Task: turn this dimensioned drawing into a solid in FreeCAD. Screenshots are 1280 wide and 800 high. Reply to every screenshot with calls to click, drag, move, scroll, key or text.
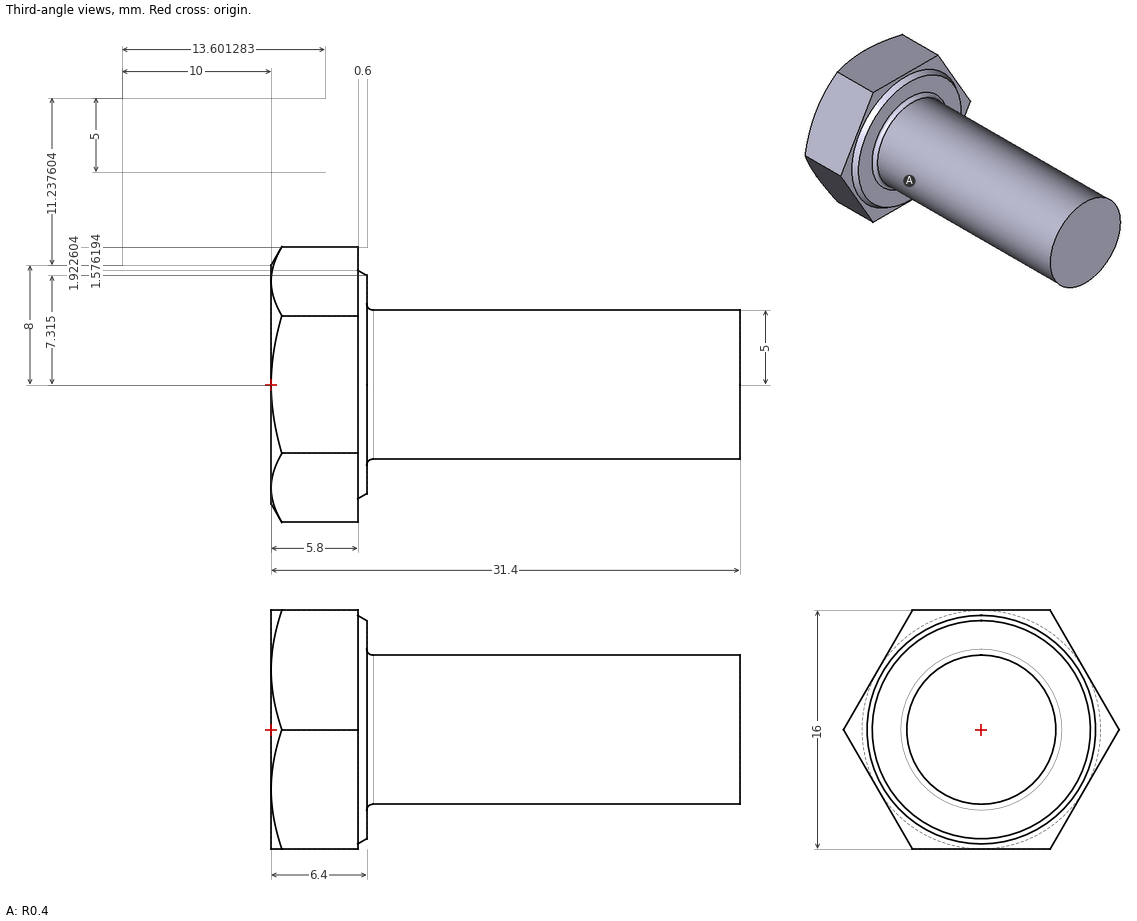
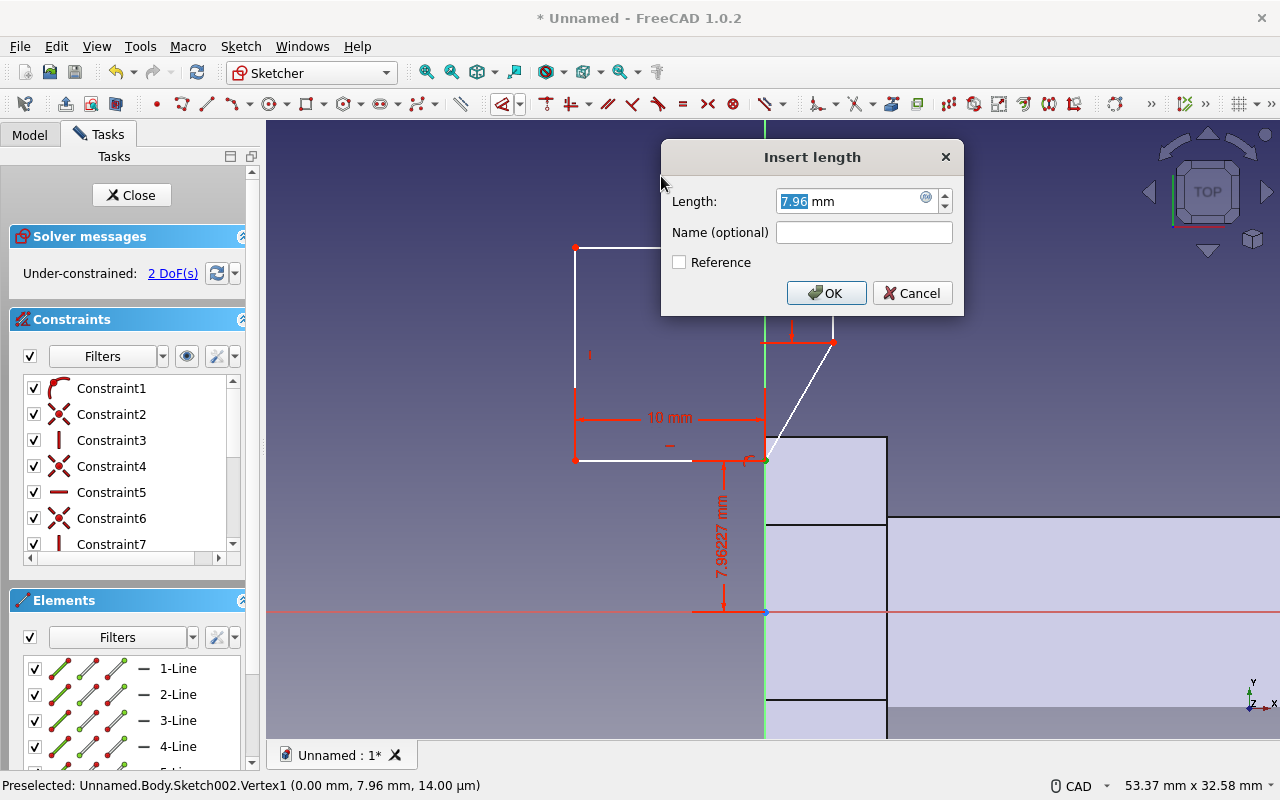
text(8)
key(Return)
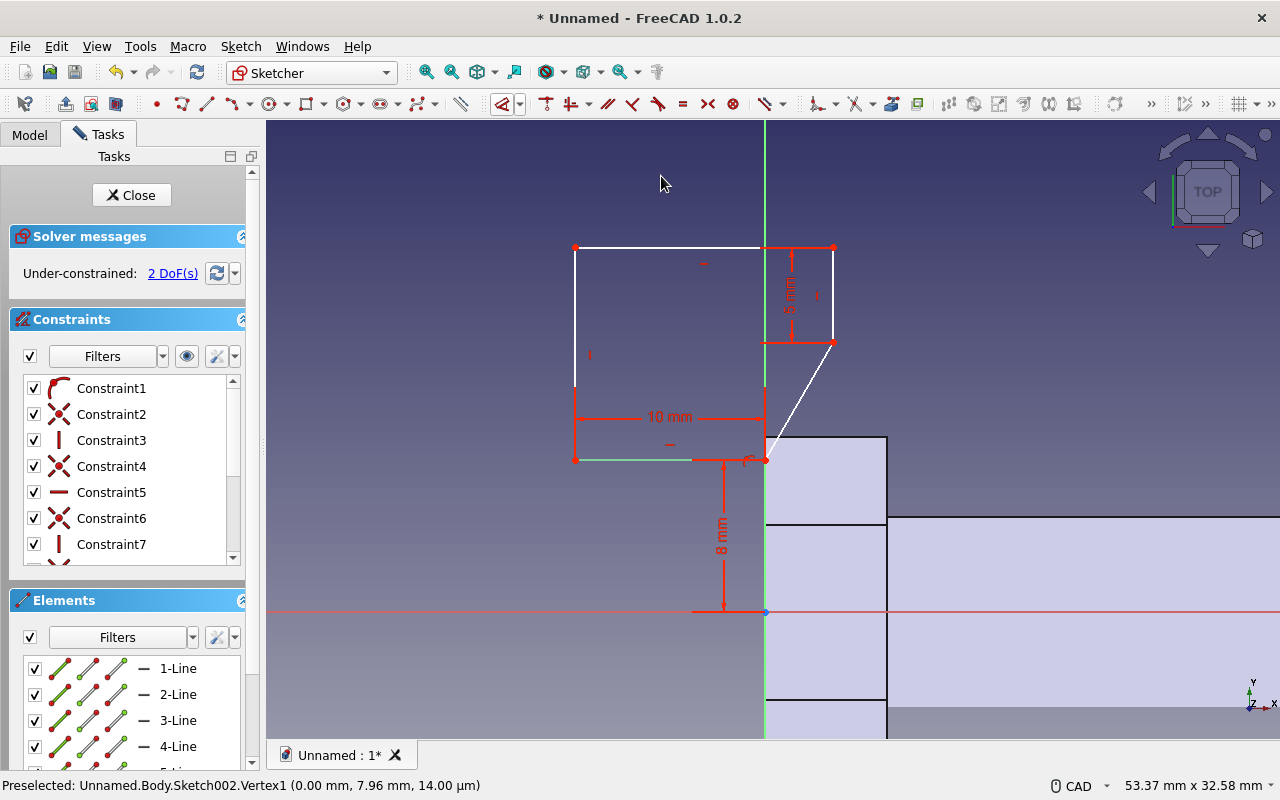
scroll(756, 248, up, 2)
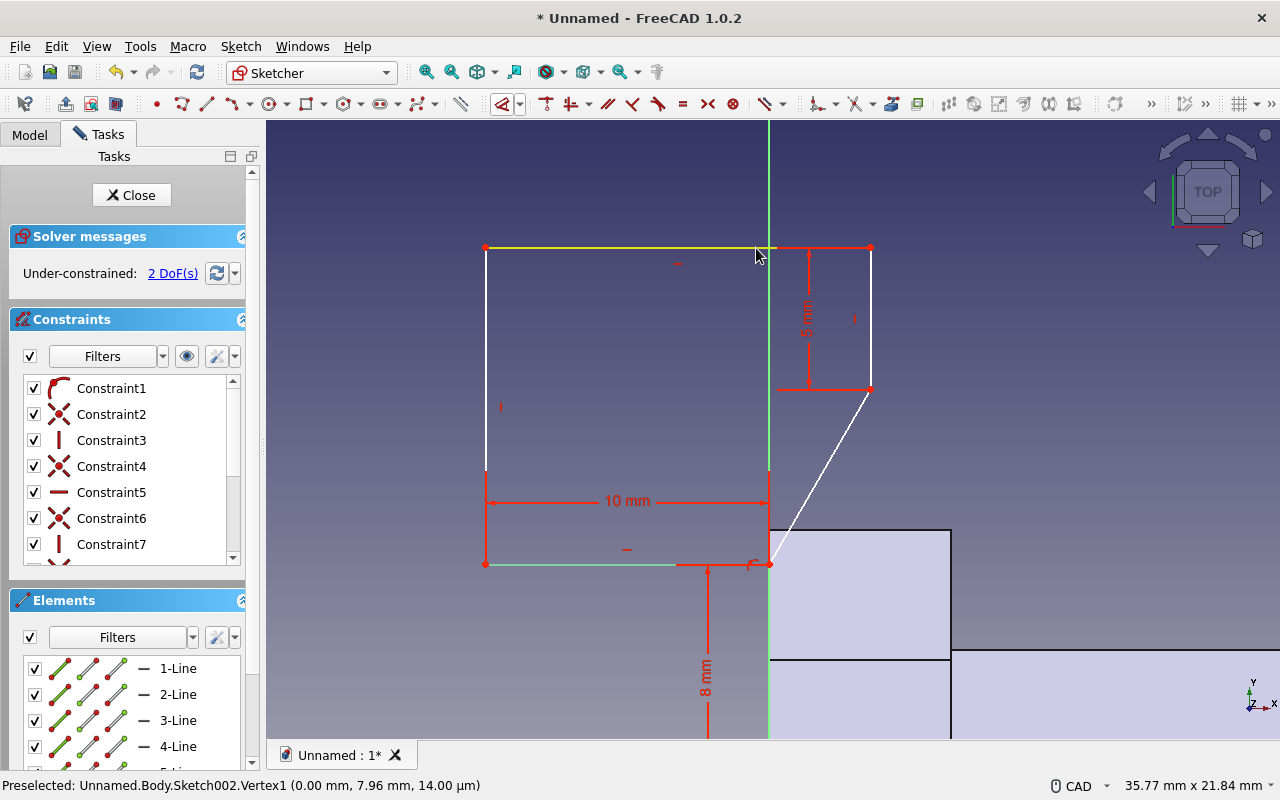
click(755, 248)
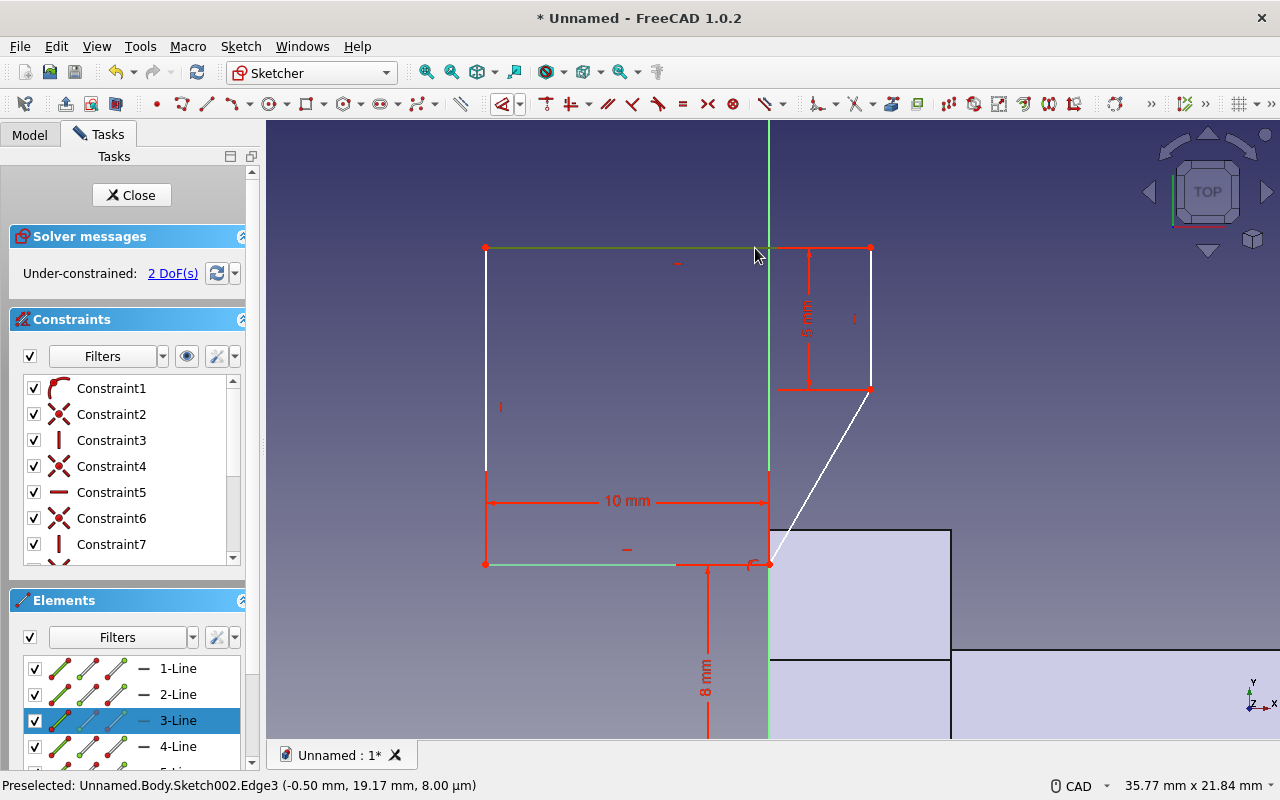
click(520, 104)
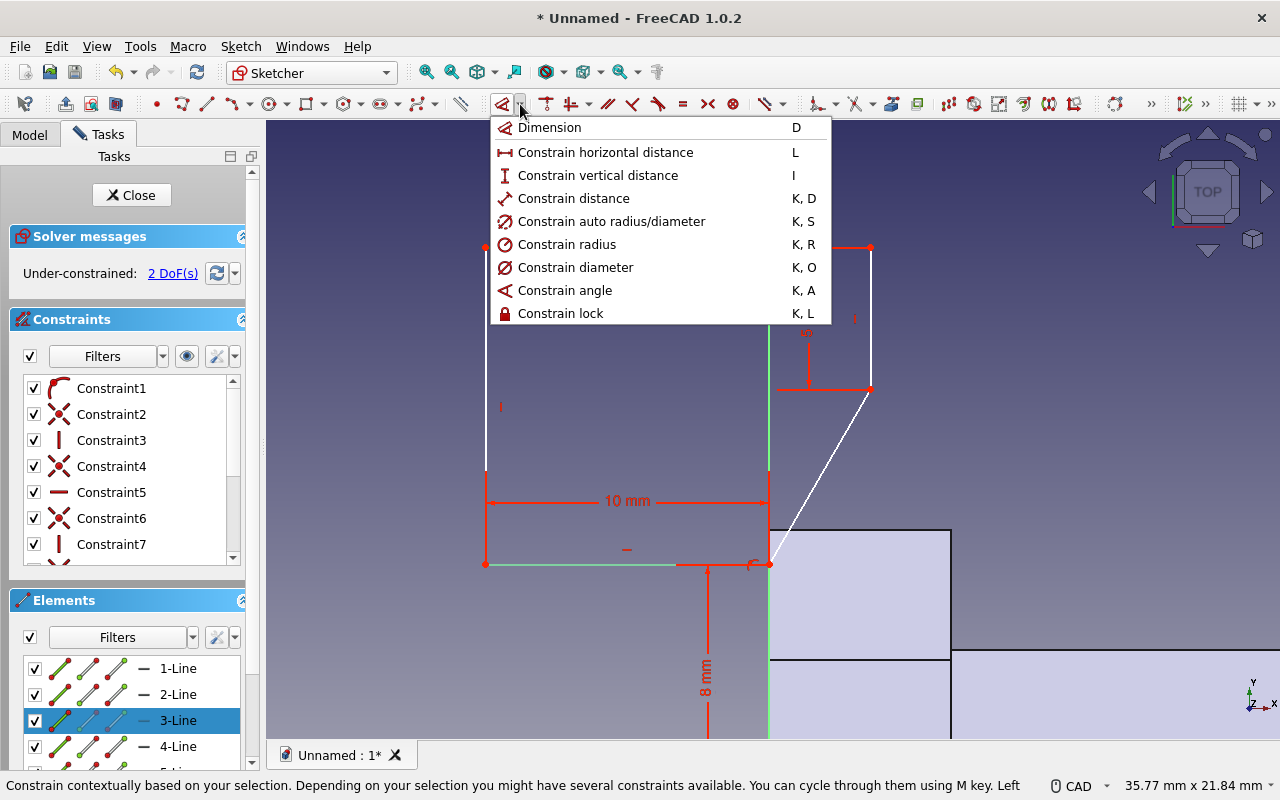
click(661, 152)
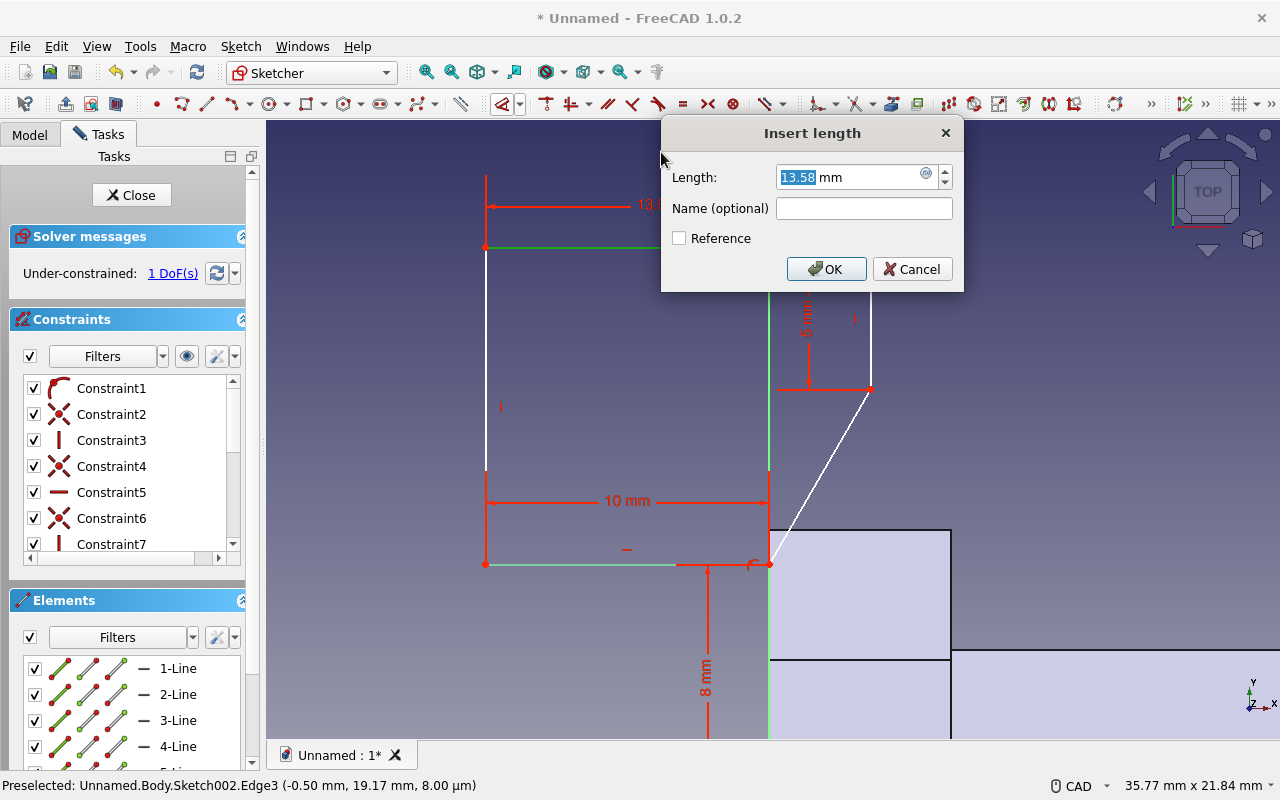
text(13.601283)
key(Return)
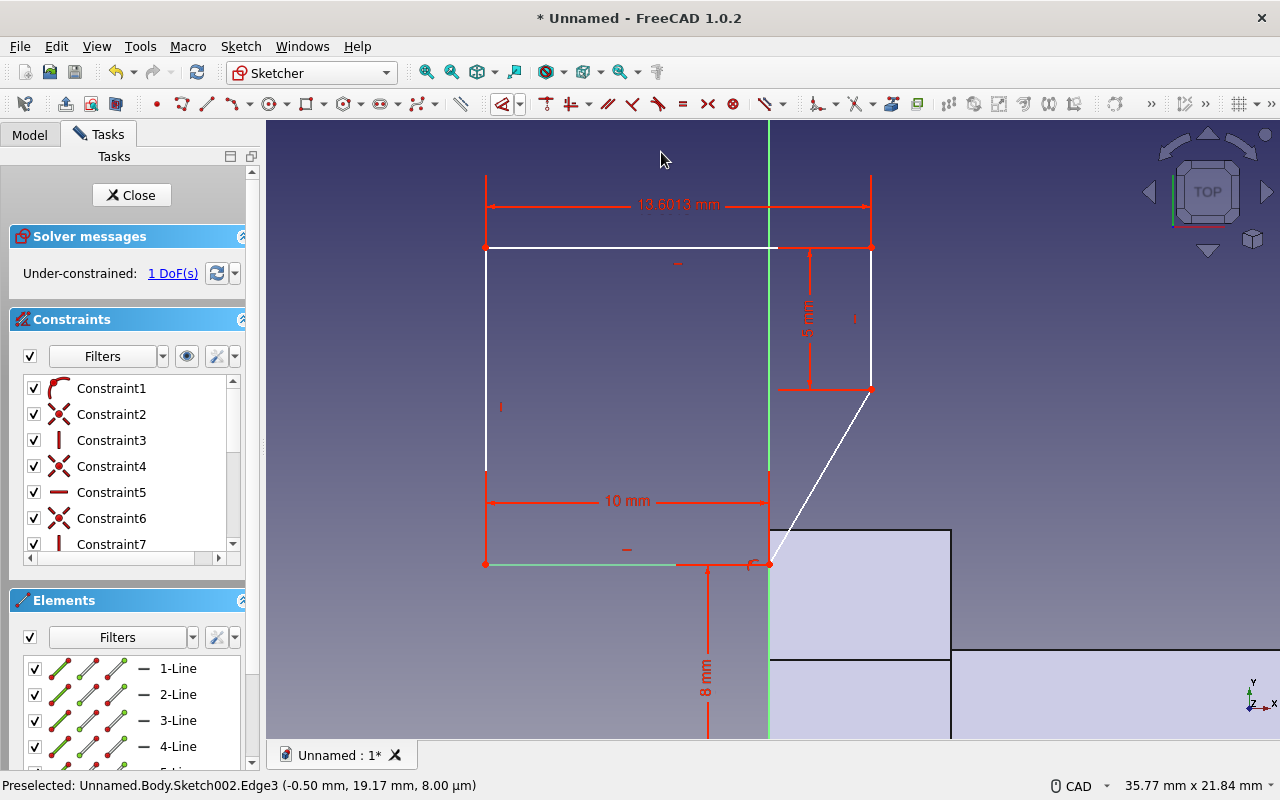
click(486, 343)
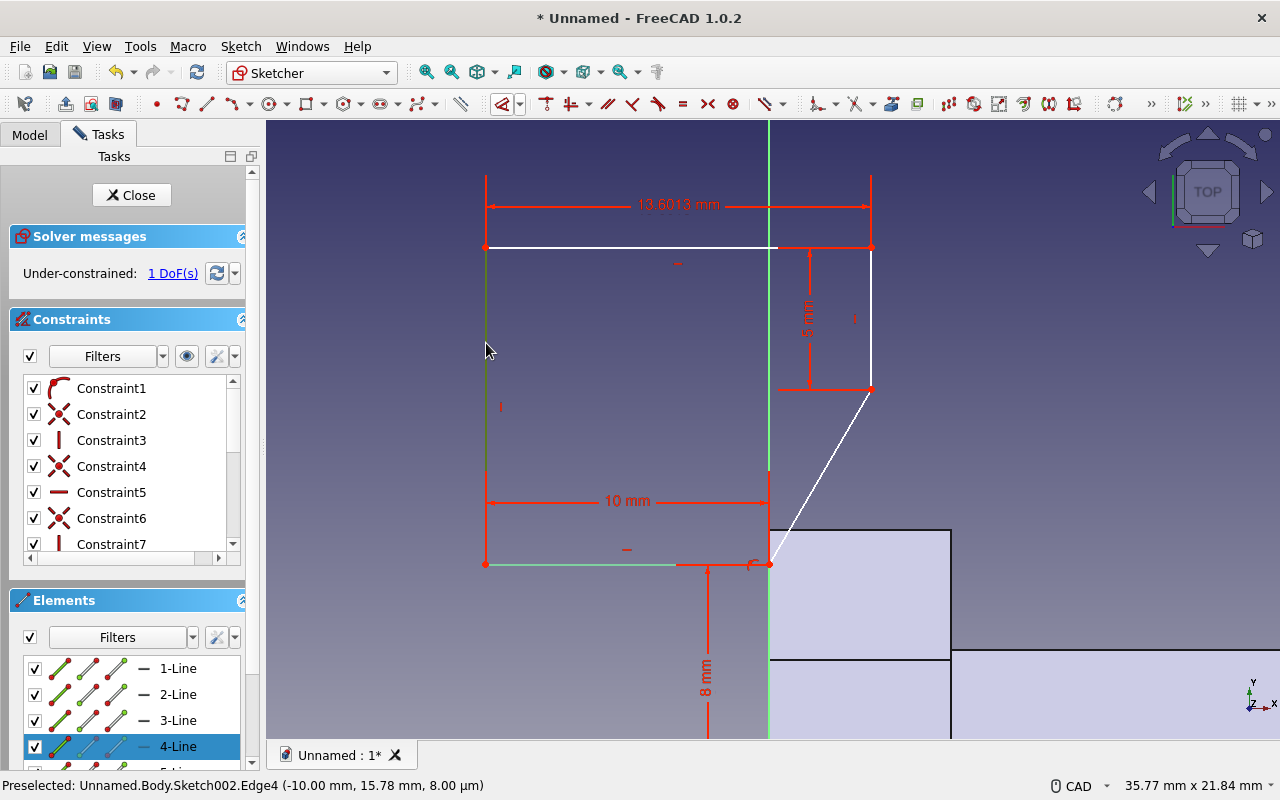
key(i)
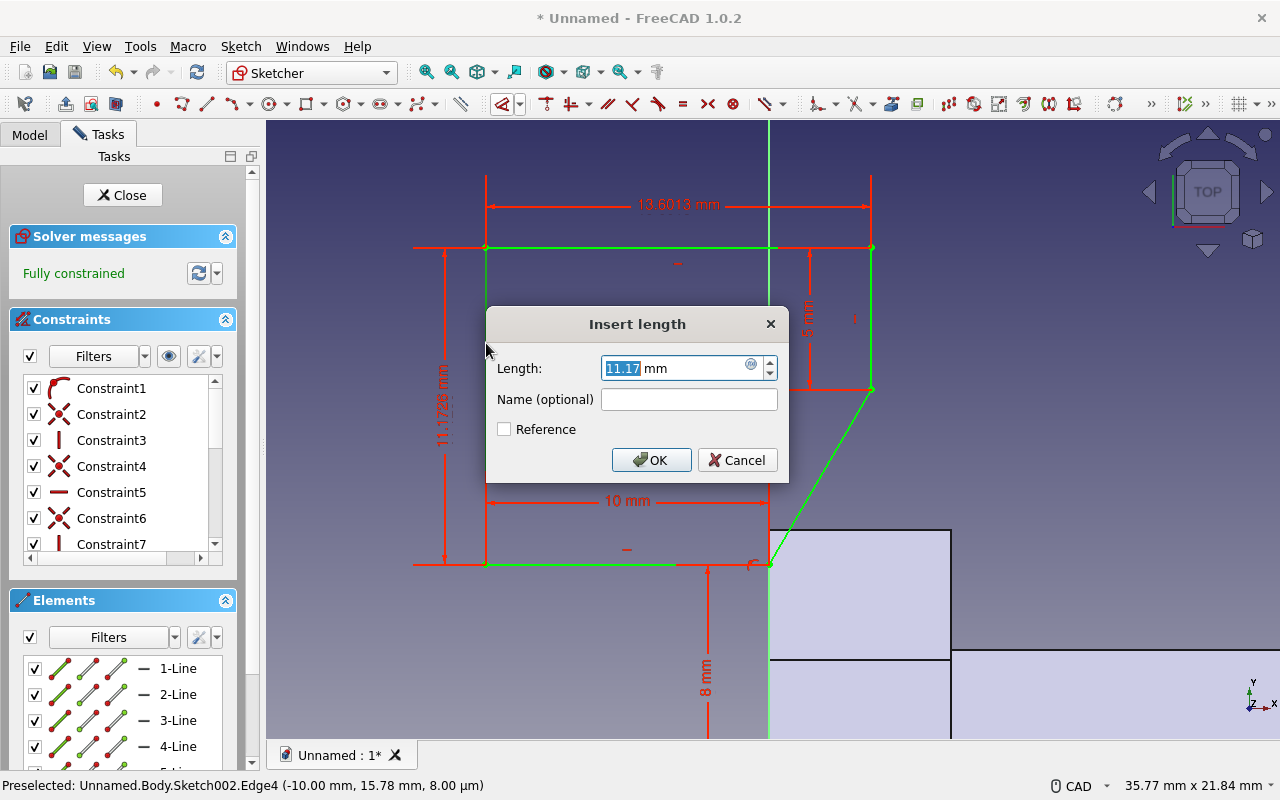
text(11.237604)
key(Return)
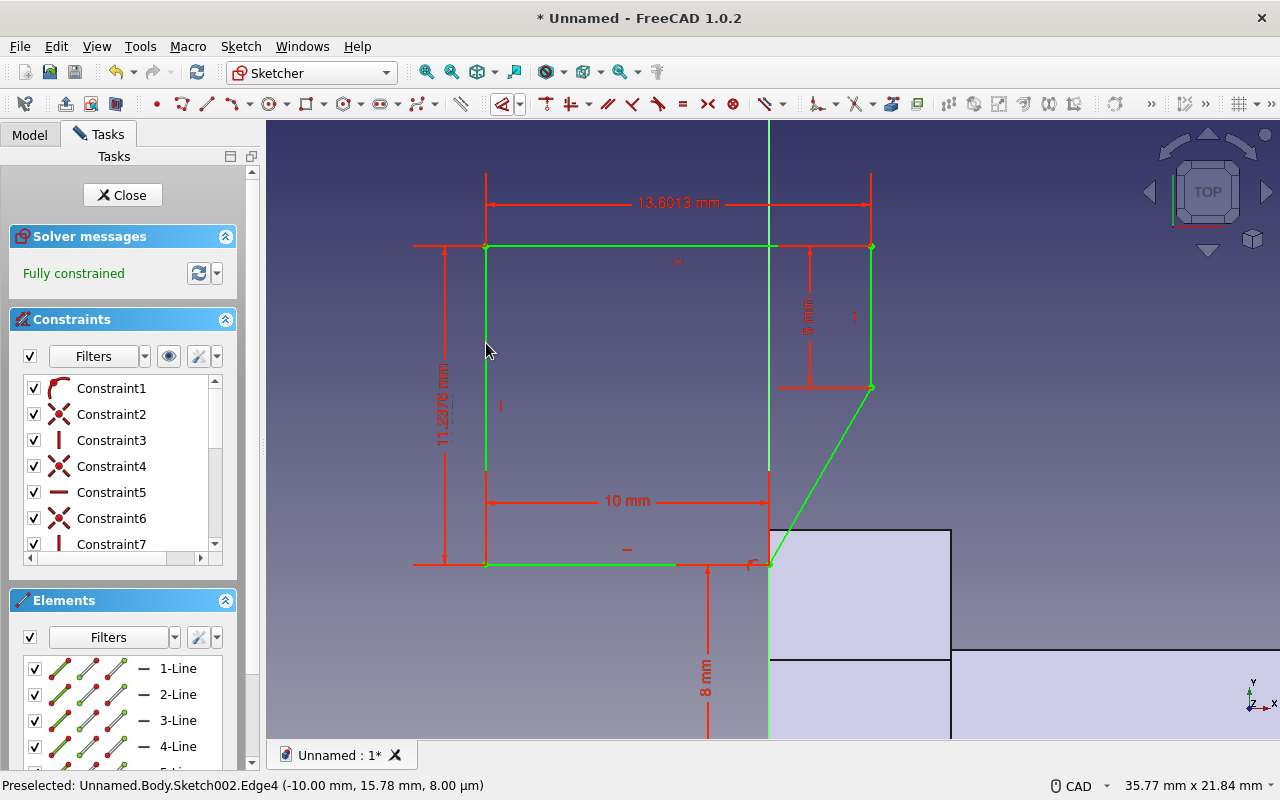
click(123, 195)